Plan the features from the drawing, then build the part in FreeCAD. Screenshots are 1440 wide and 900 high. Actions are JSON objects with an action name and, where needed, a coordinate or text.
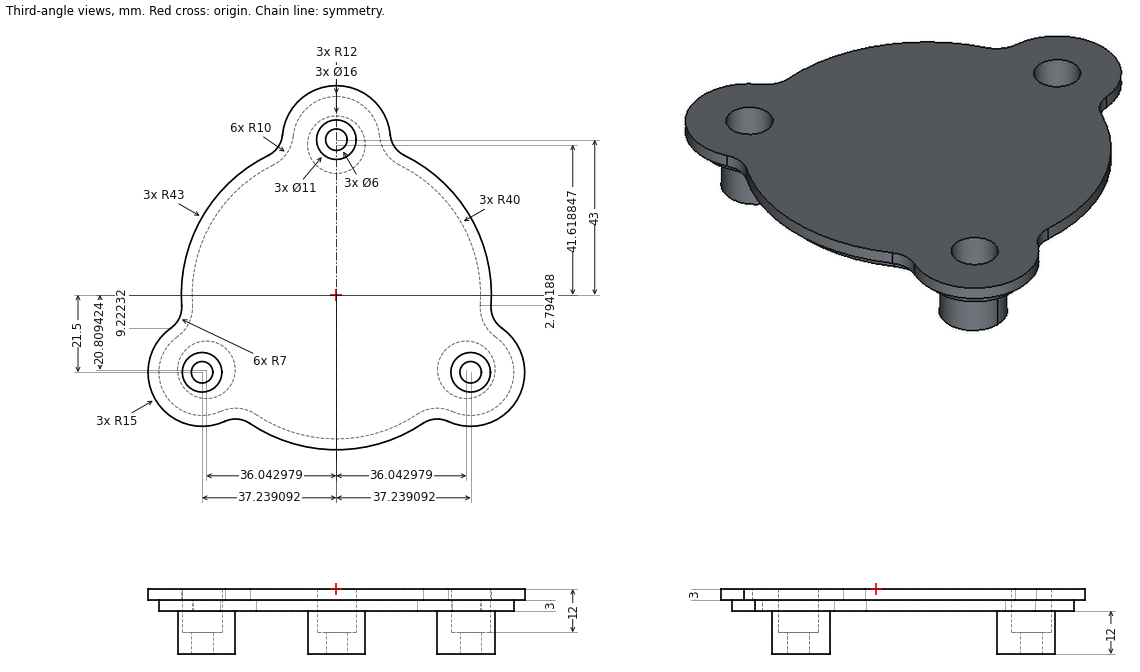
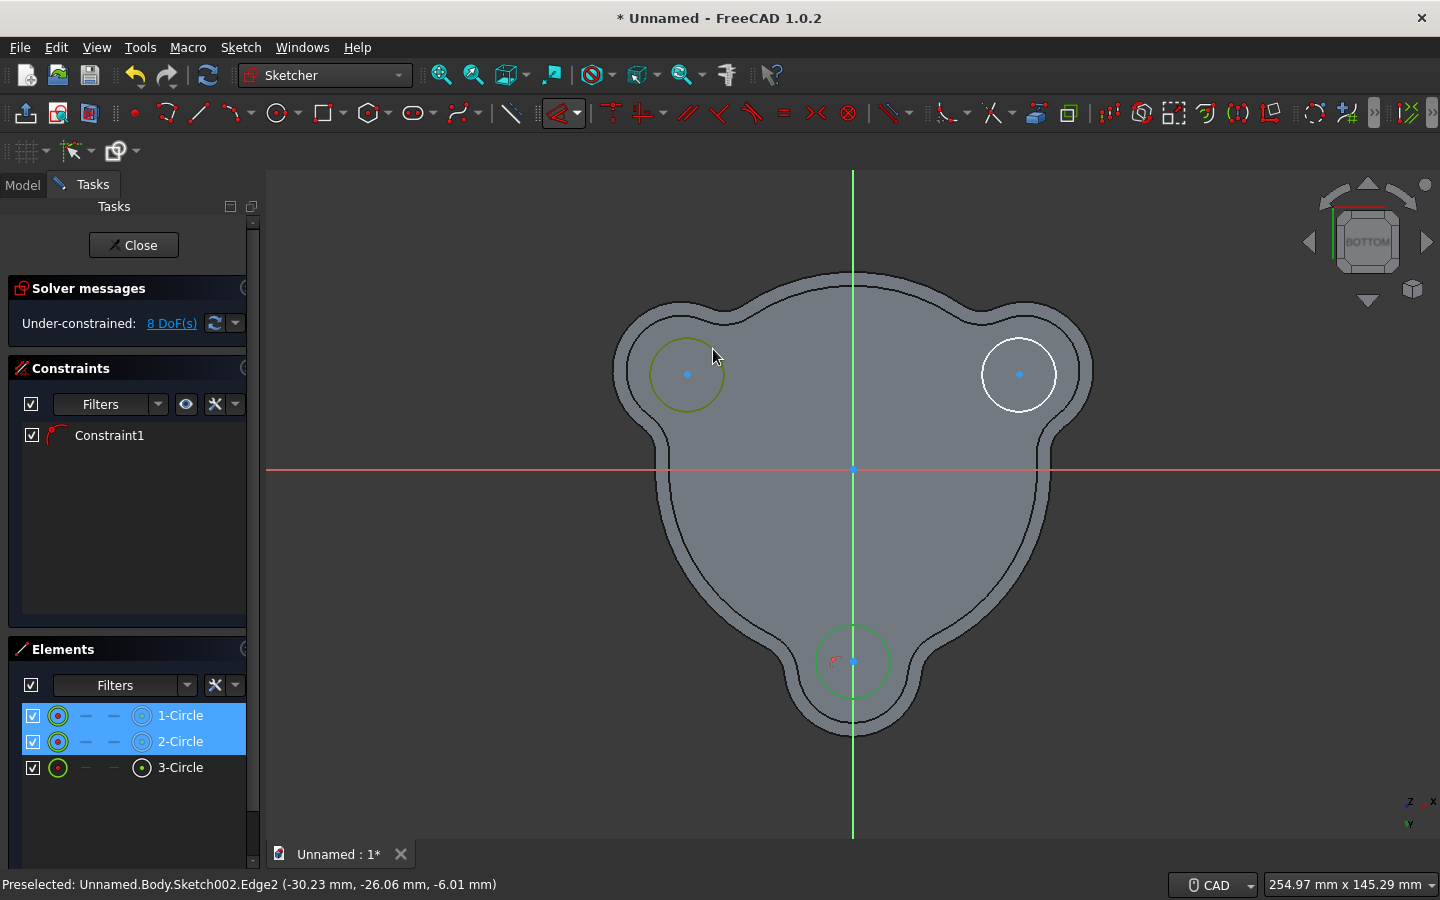
{"action": "left_click", "coordinate": [1045, 349]}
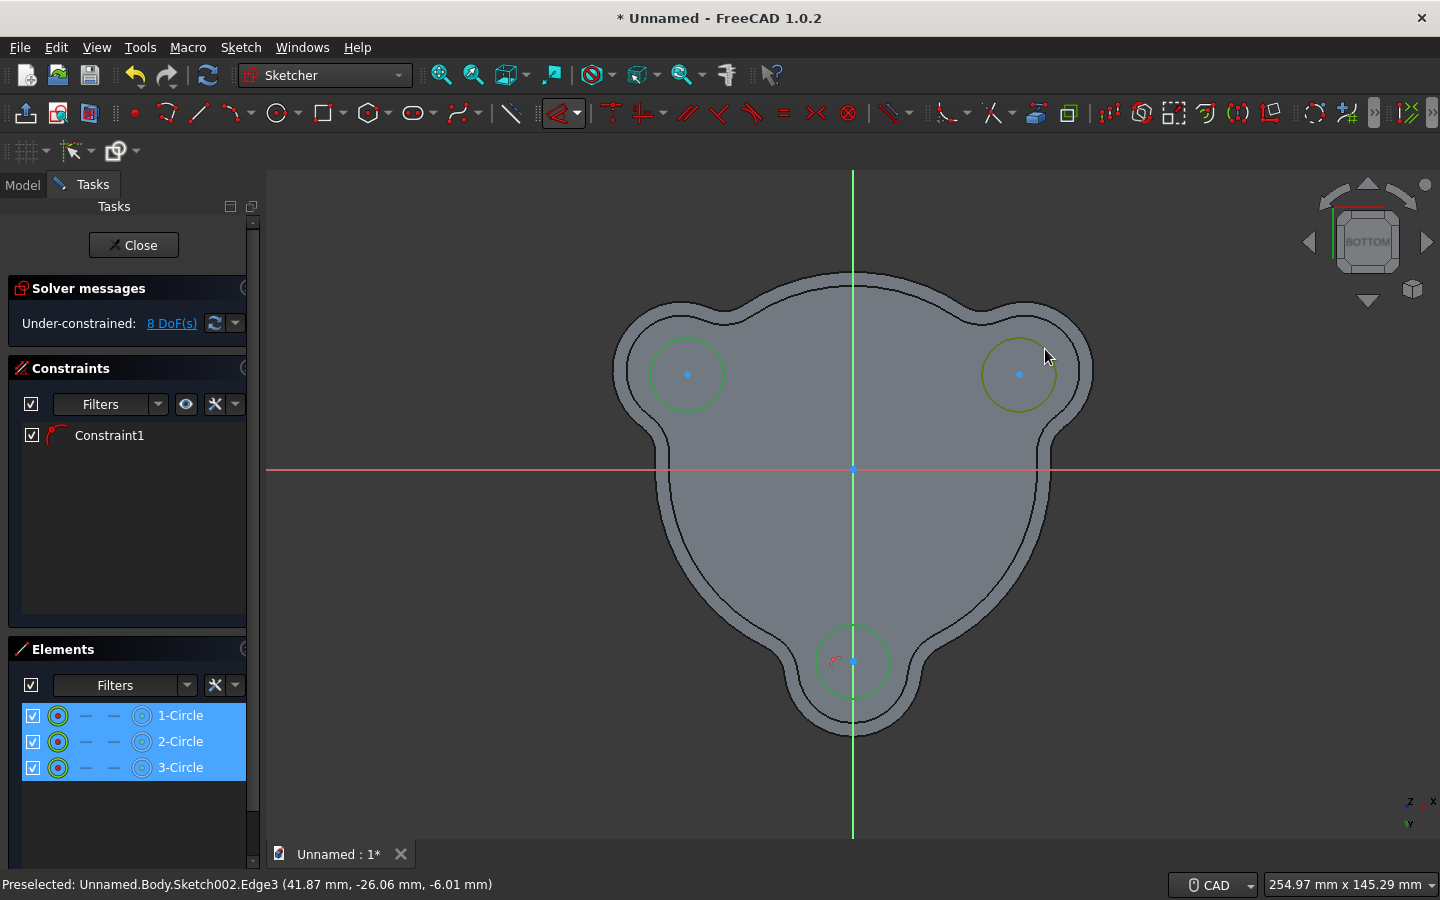
{"action": "left_click", "coordinate": [784, 114]}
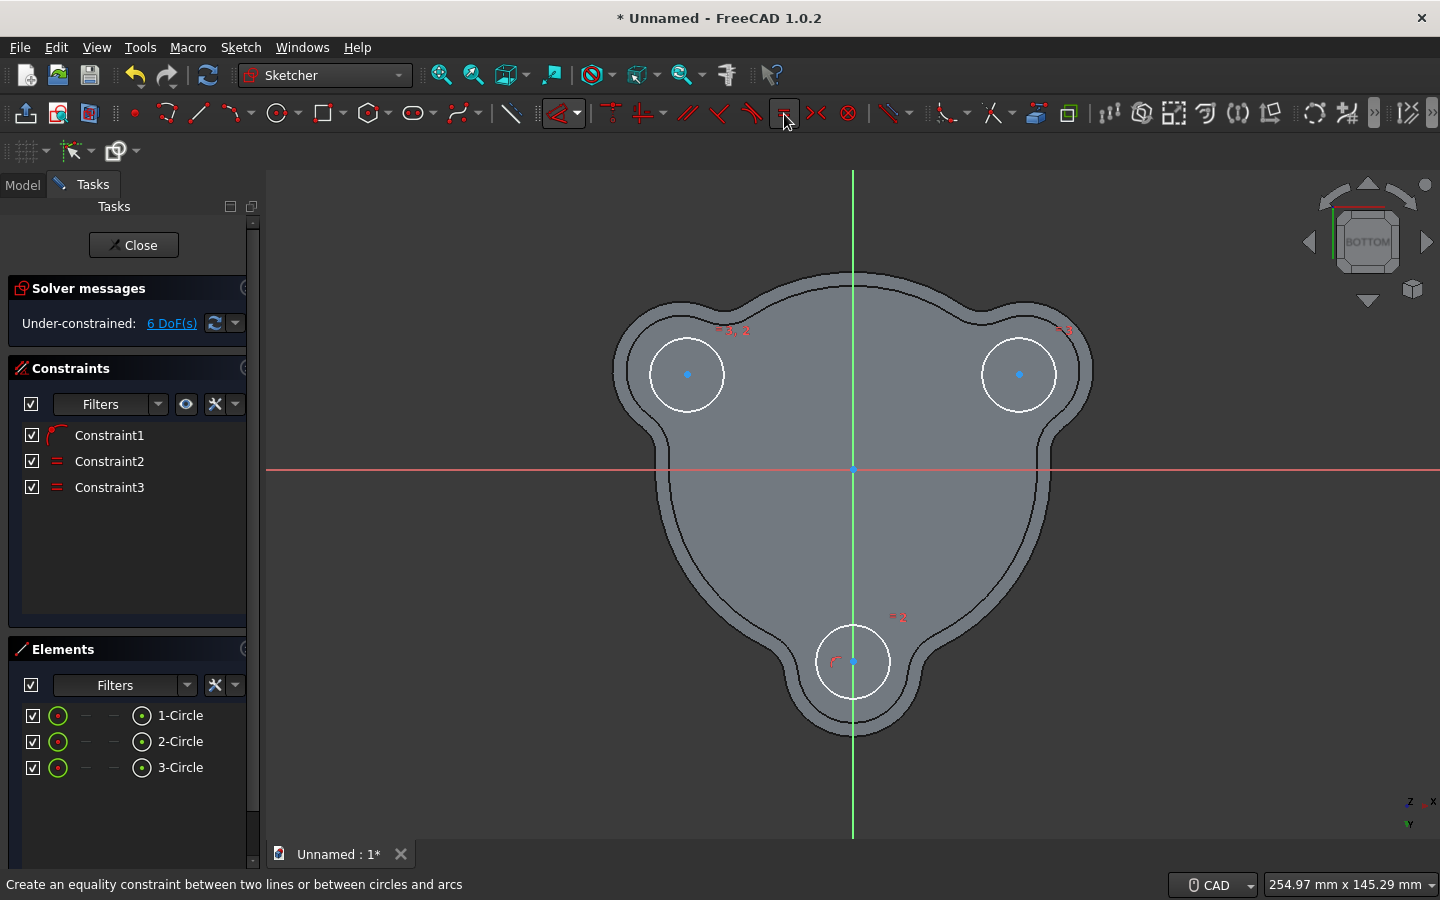
{"action": "left_click", "coordinate": [687, 375]}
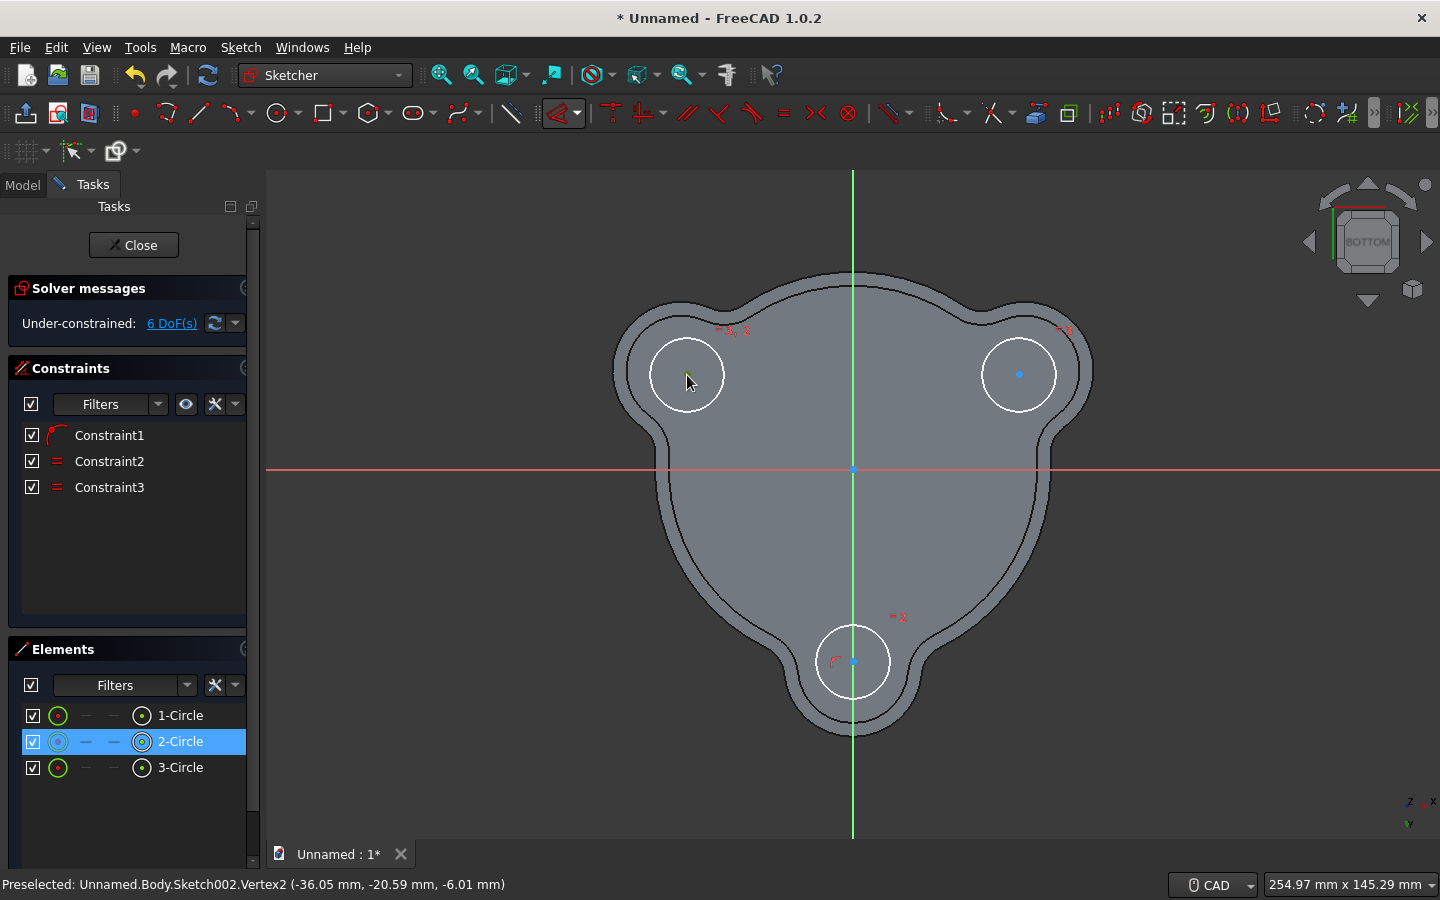
{"action": "left_click", "coordinate": [1019, 375]}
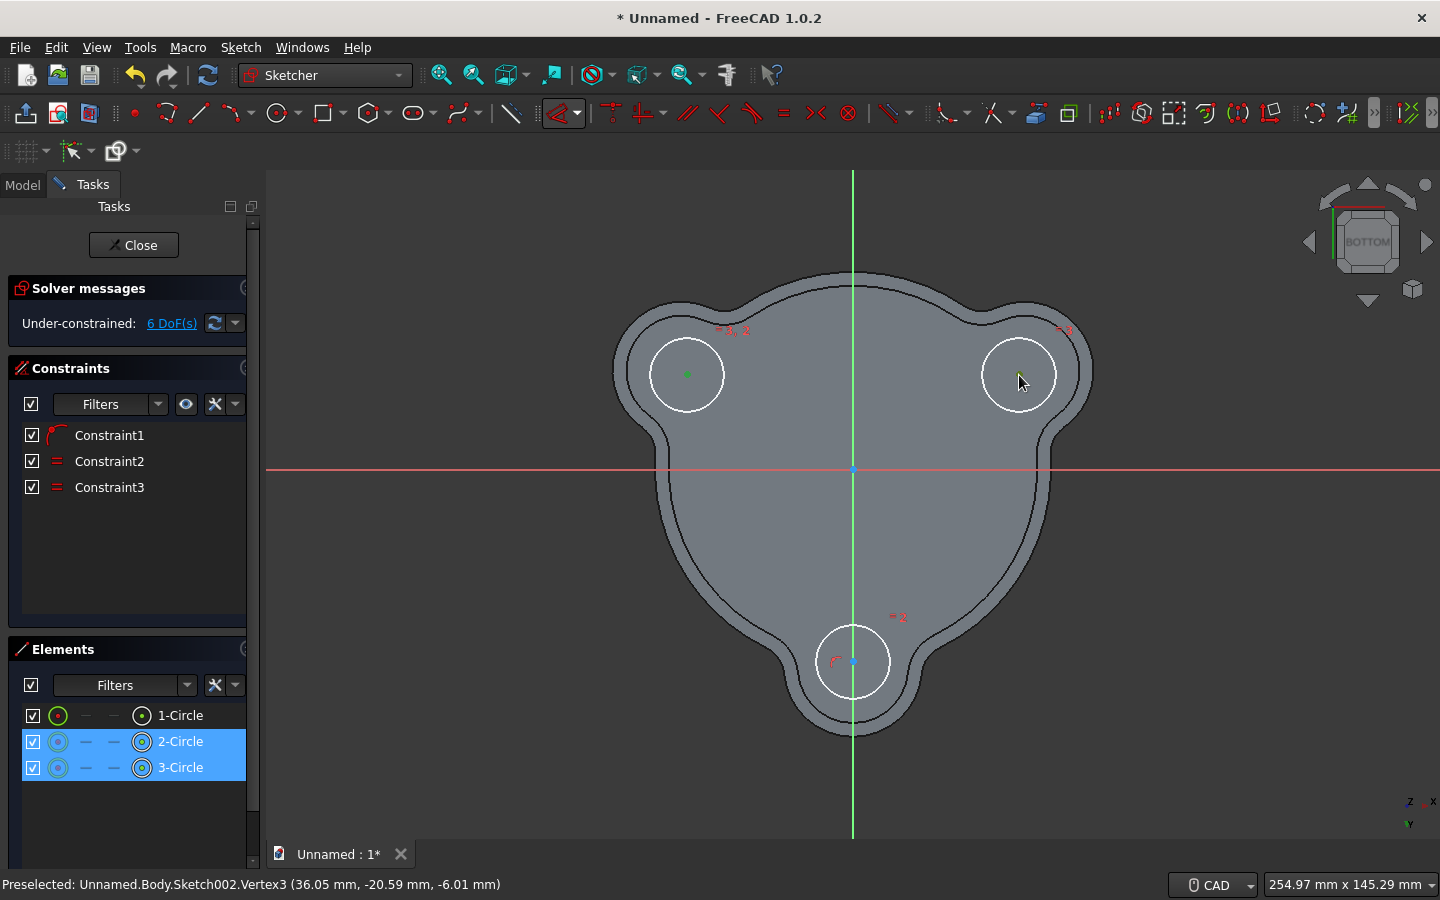
{"action": "left_click", "coordinate": [666, 114]}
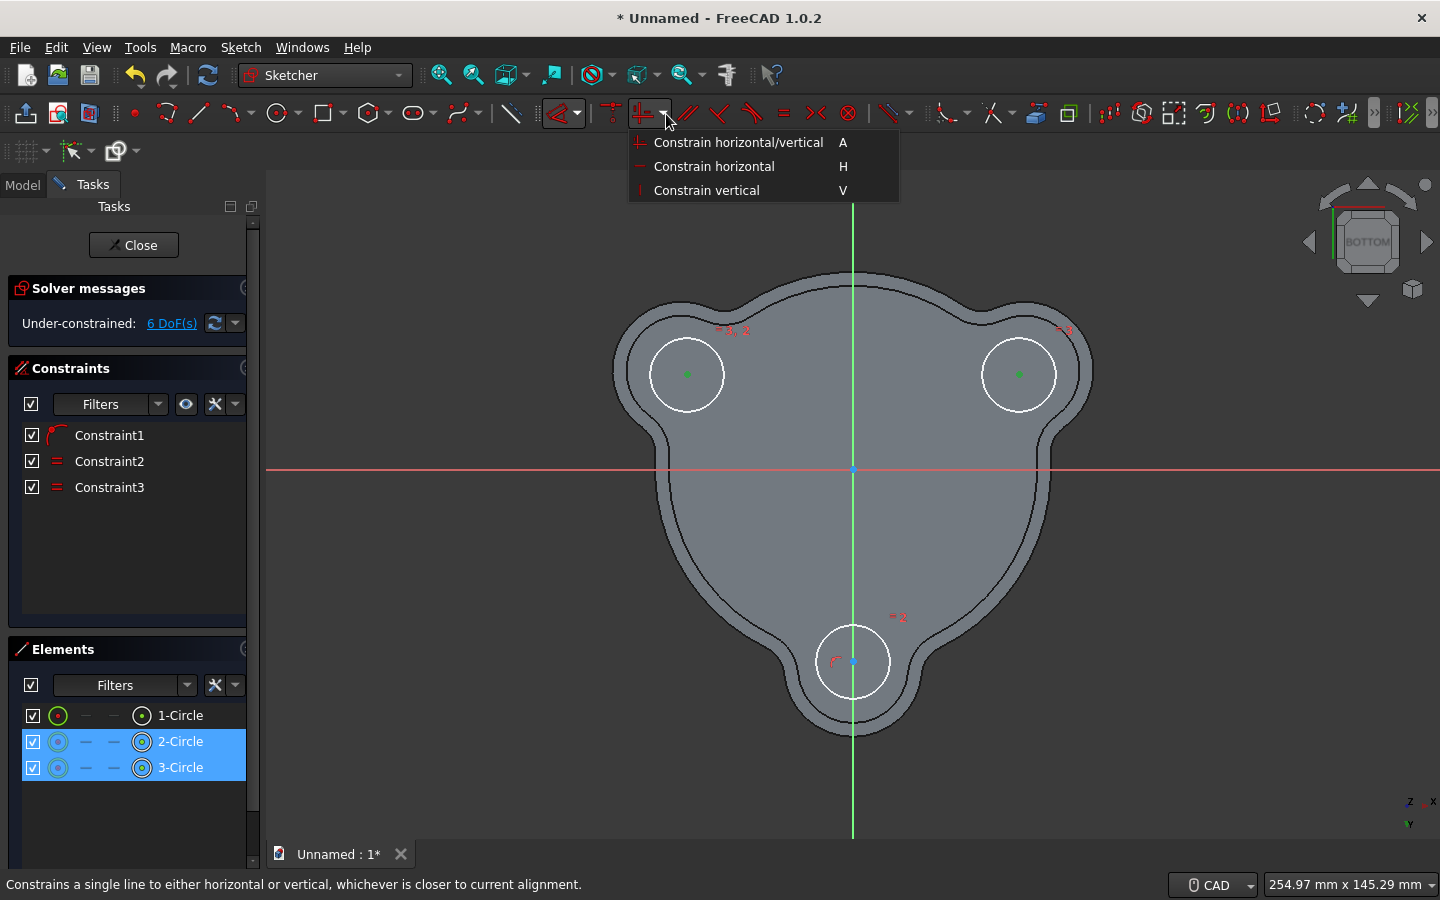
{"action": "left_click", "coordinate": [764, 166]}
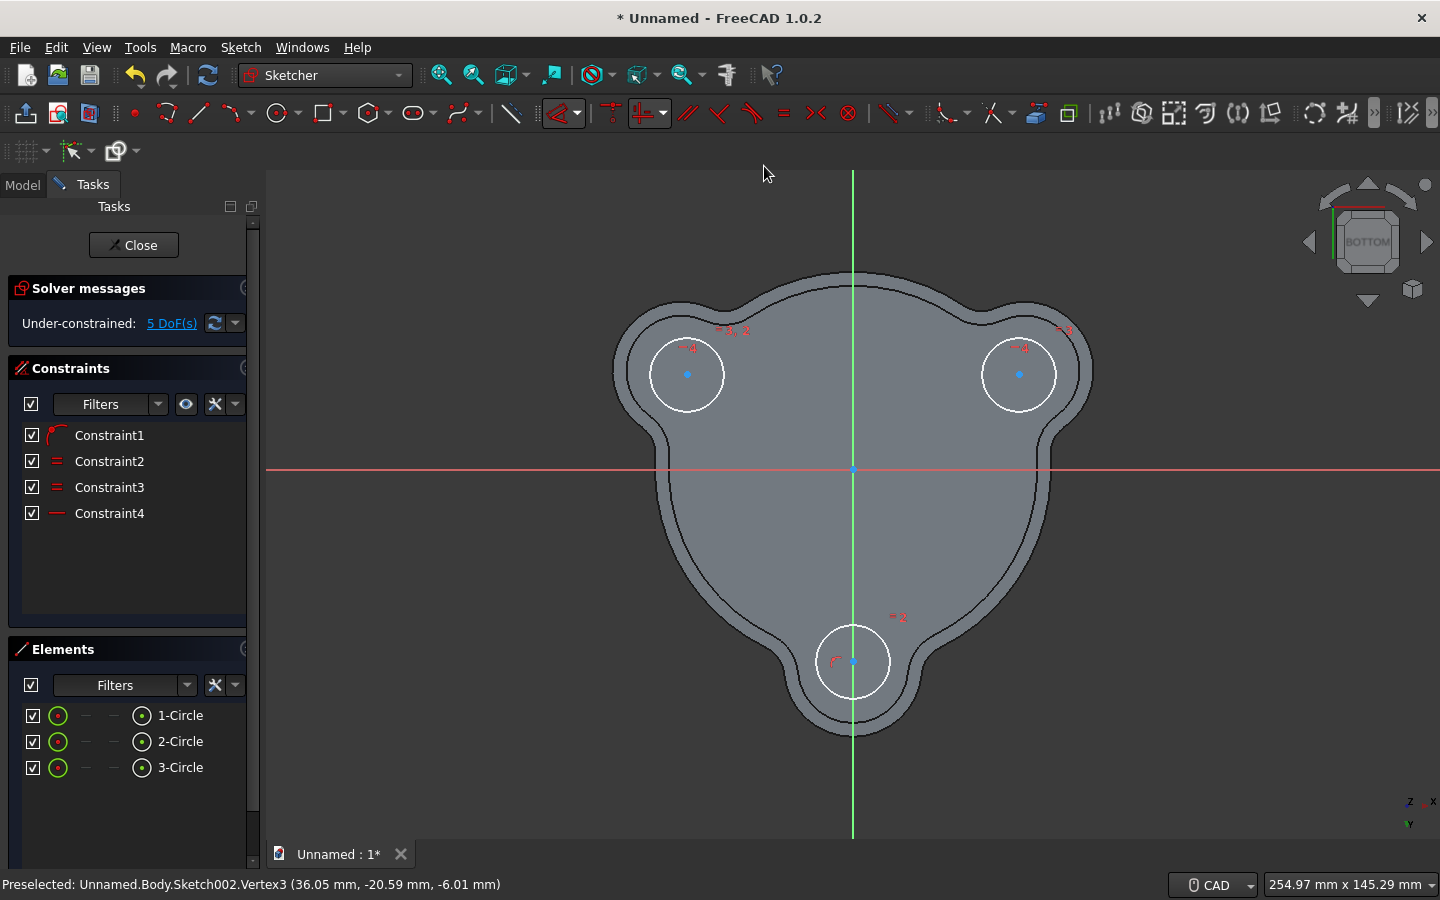
{"action": "left_click", "coordinate": [879, 636]}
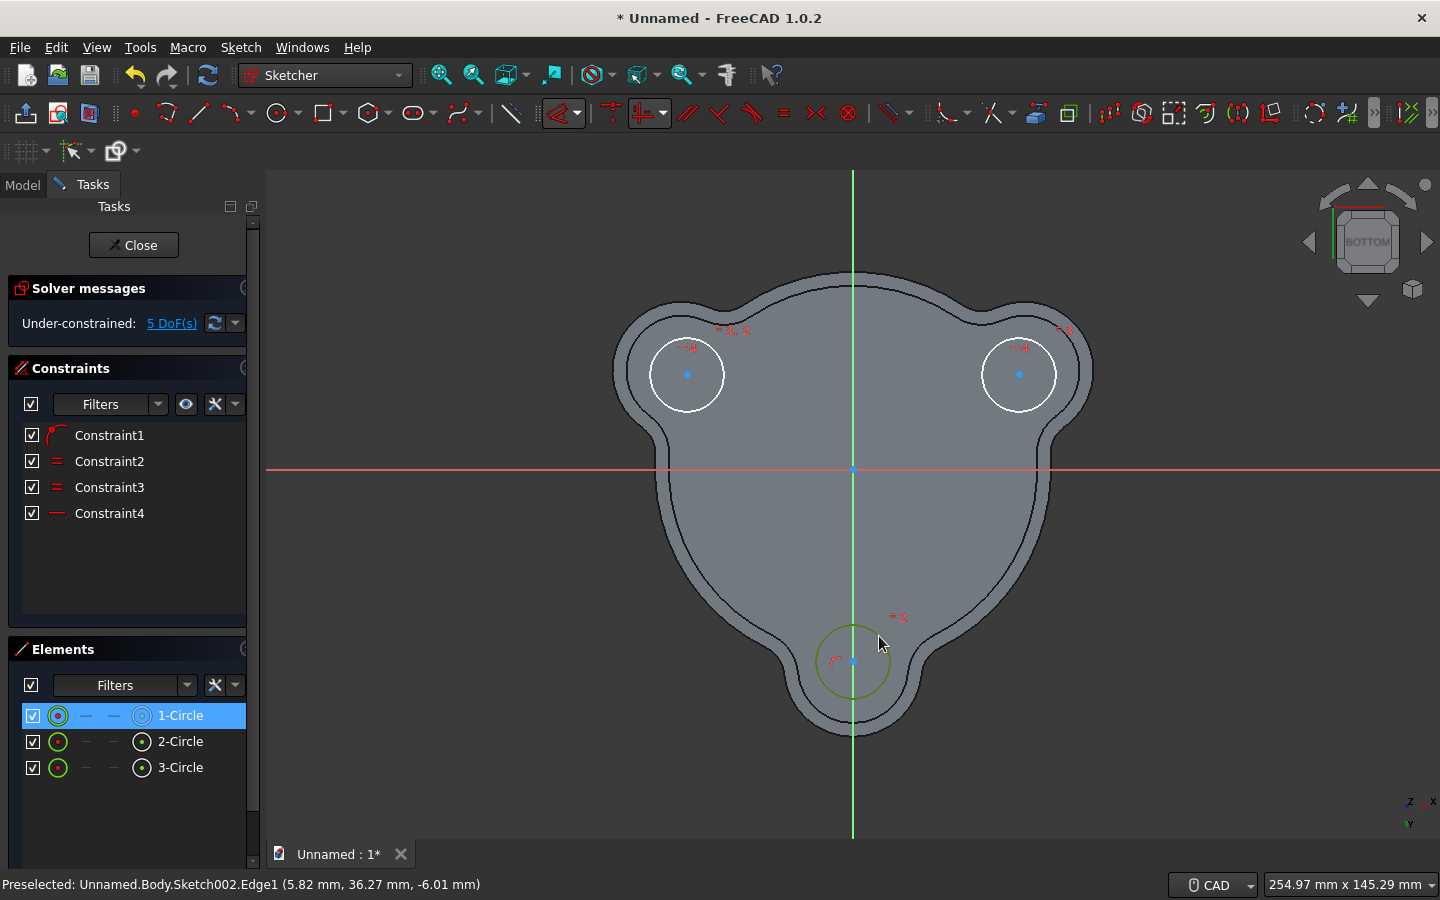
{"action": "key", "text": "k o"}